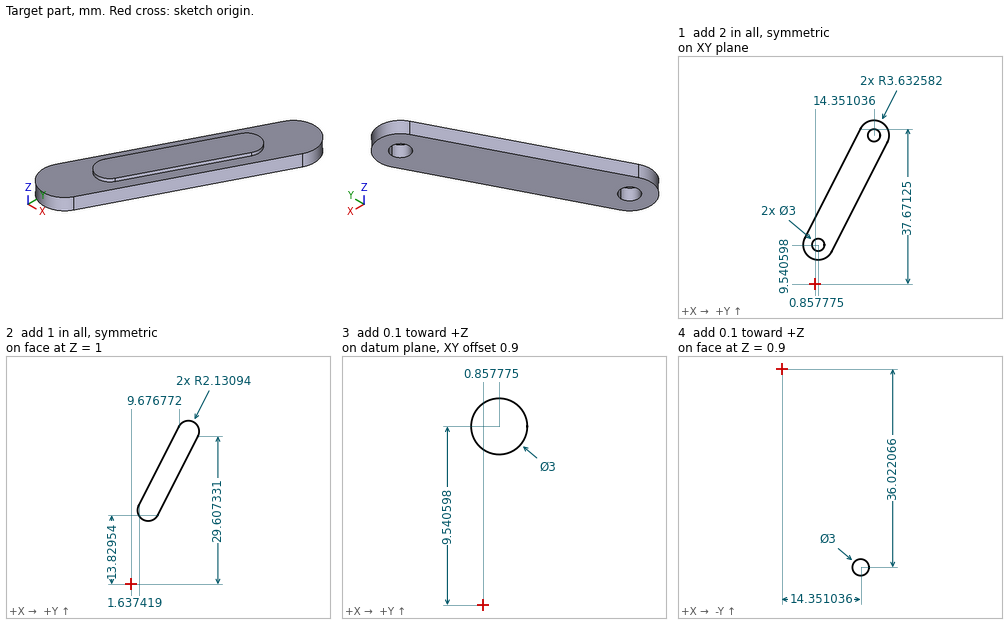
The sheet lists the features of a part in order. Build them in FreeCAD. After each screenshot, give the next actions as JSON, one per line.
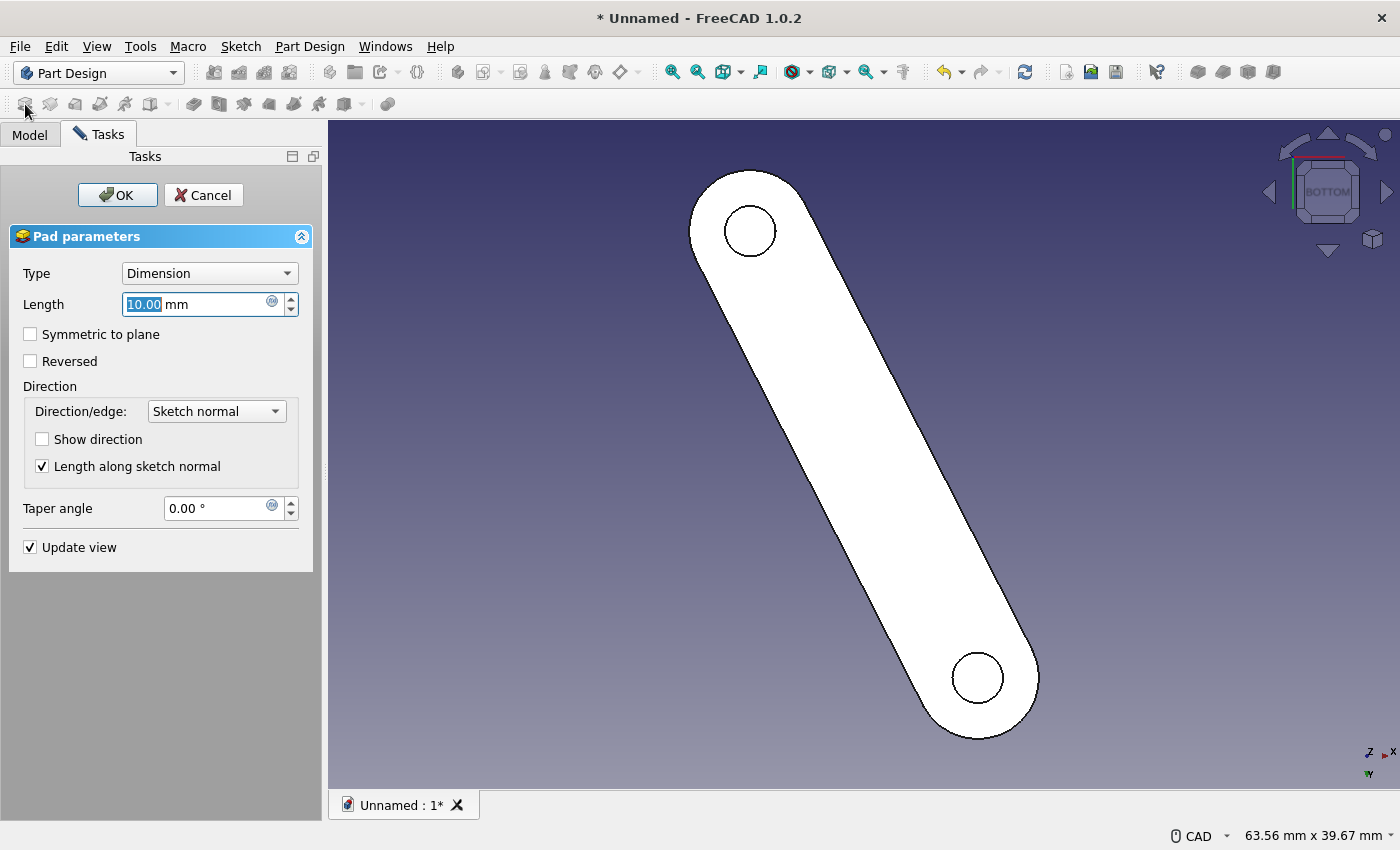
{"action": "type", "text": "0.1"}
{"action": "key", "text": "Tab"}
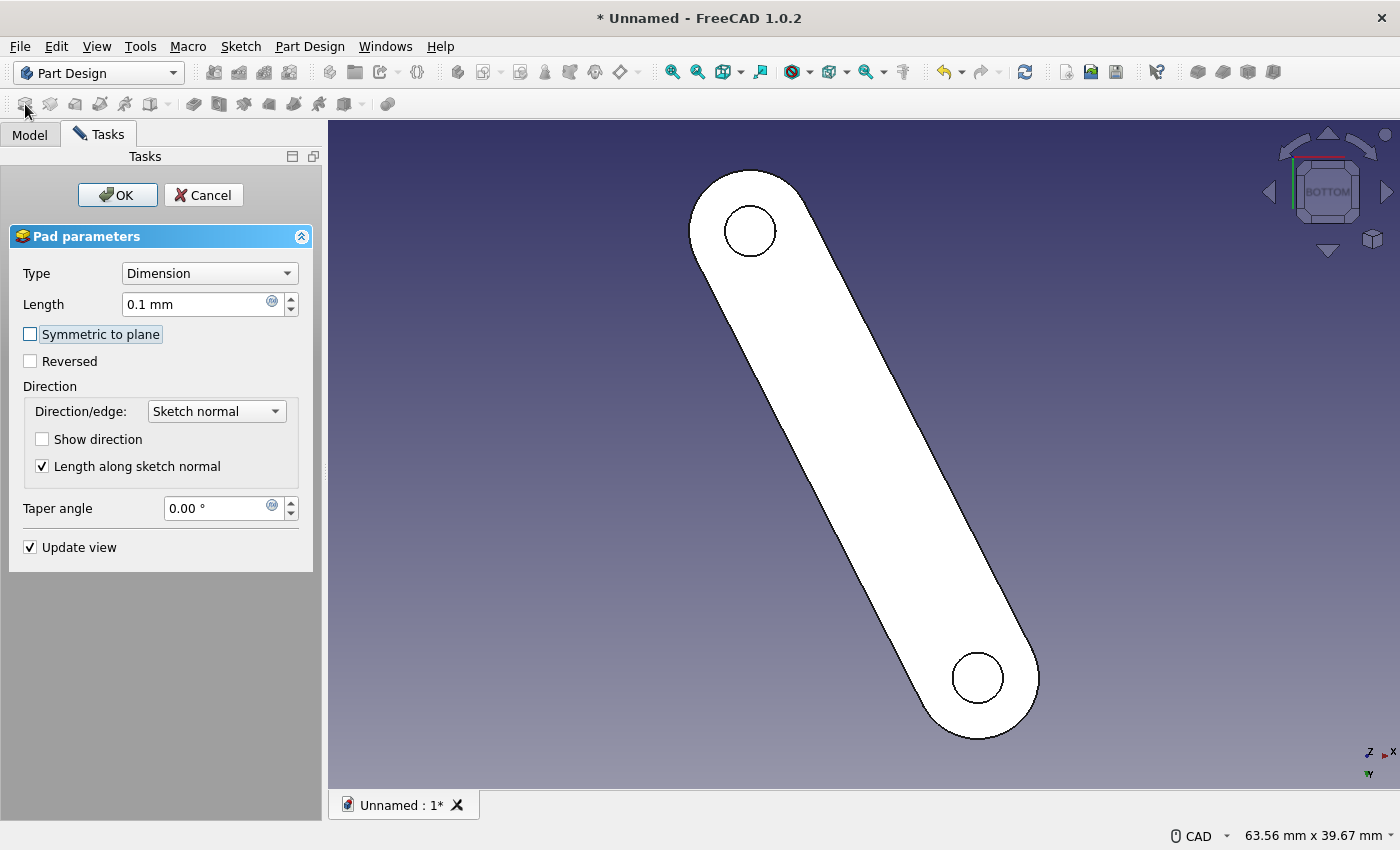
{"action": "left_click", "coordinate": [31, 361]}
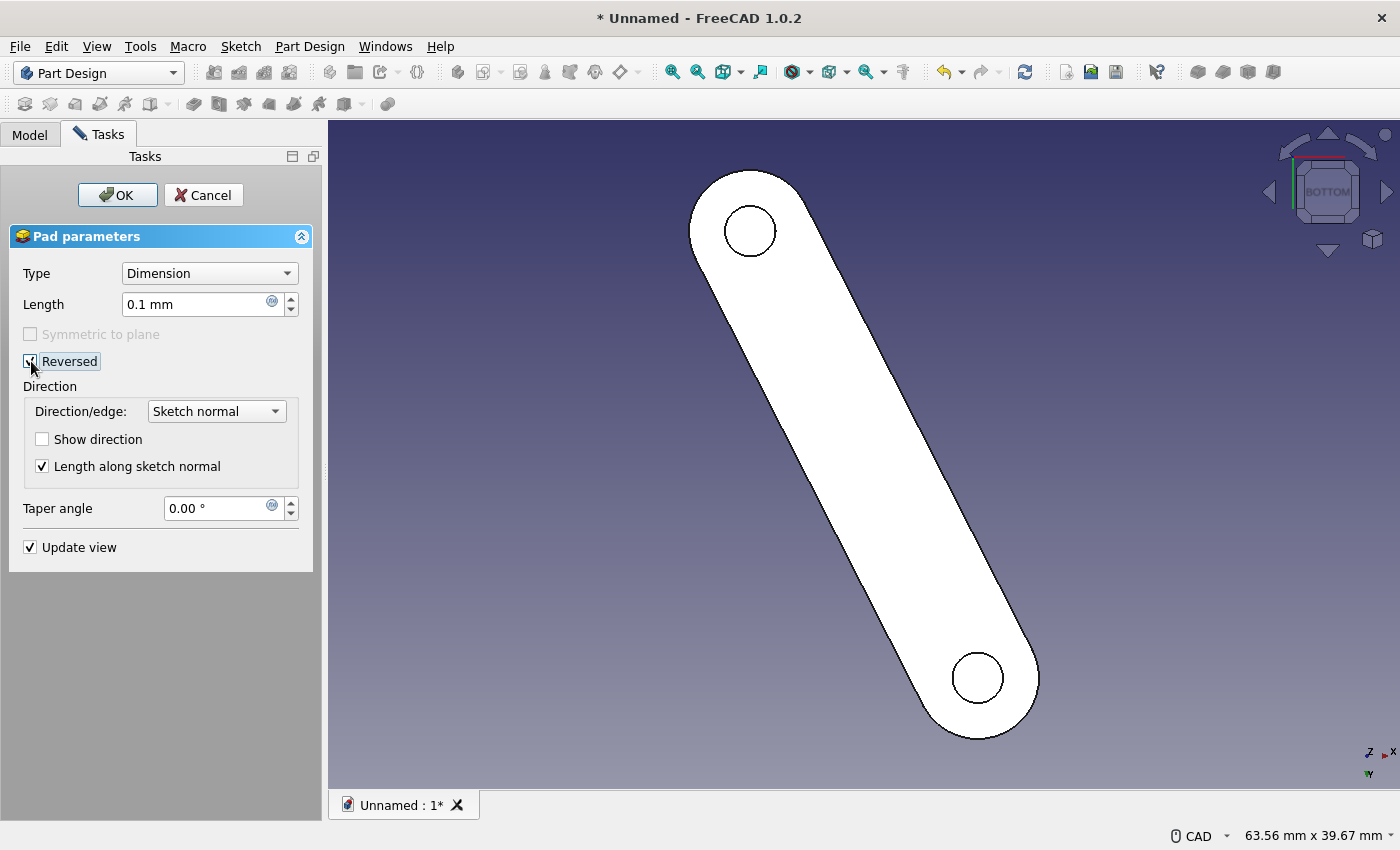
{"action": "left_click", "coordinate": [118, 195]}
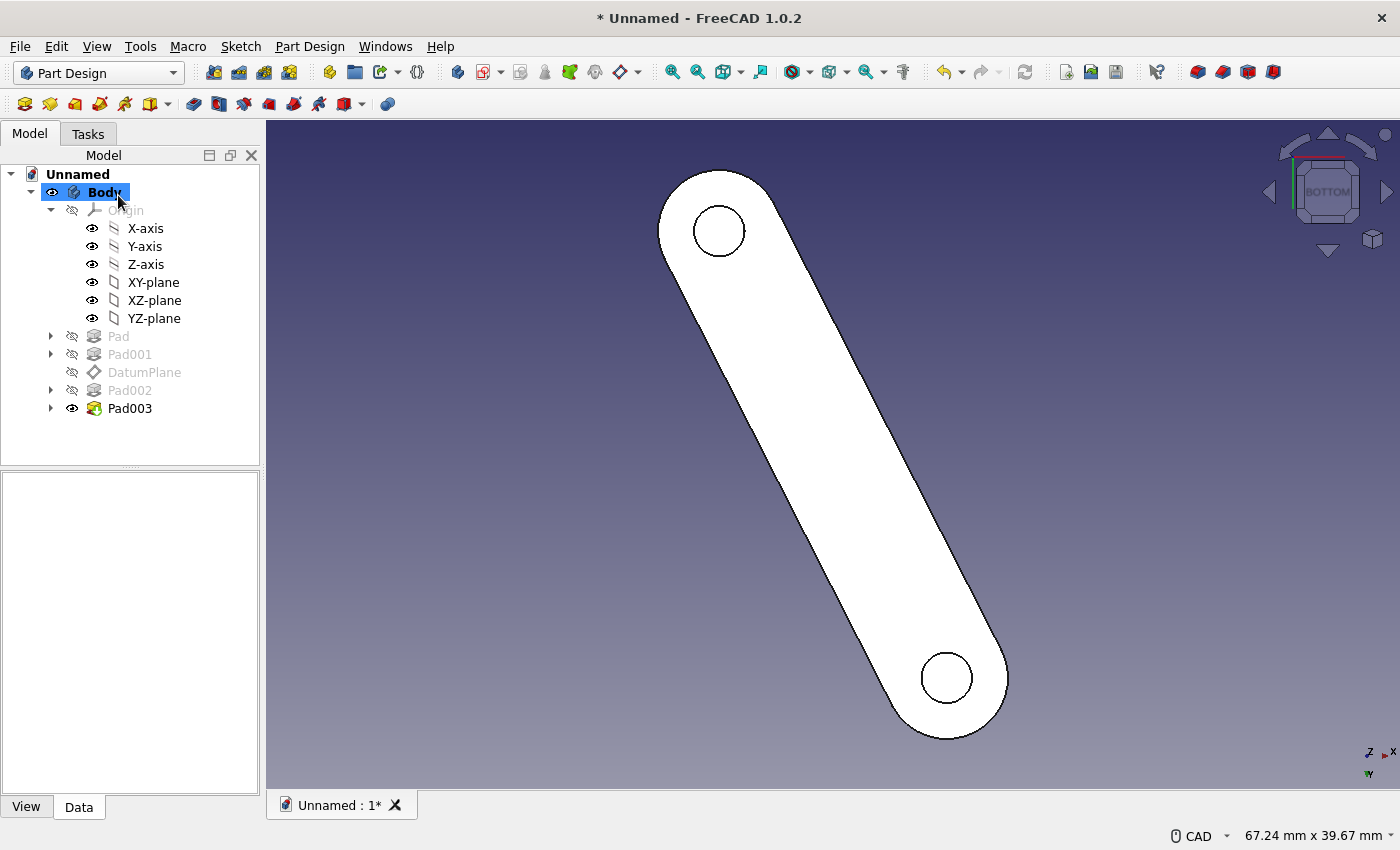
{"action": "key", "text": "0"}